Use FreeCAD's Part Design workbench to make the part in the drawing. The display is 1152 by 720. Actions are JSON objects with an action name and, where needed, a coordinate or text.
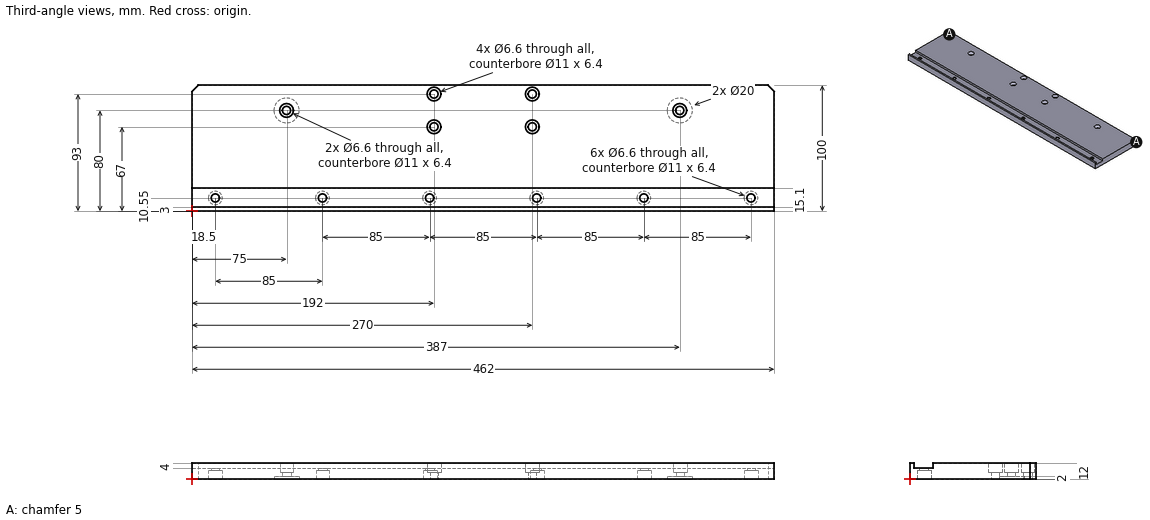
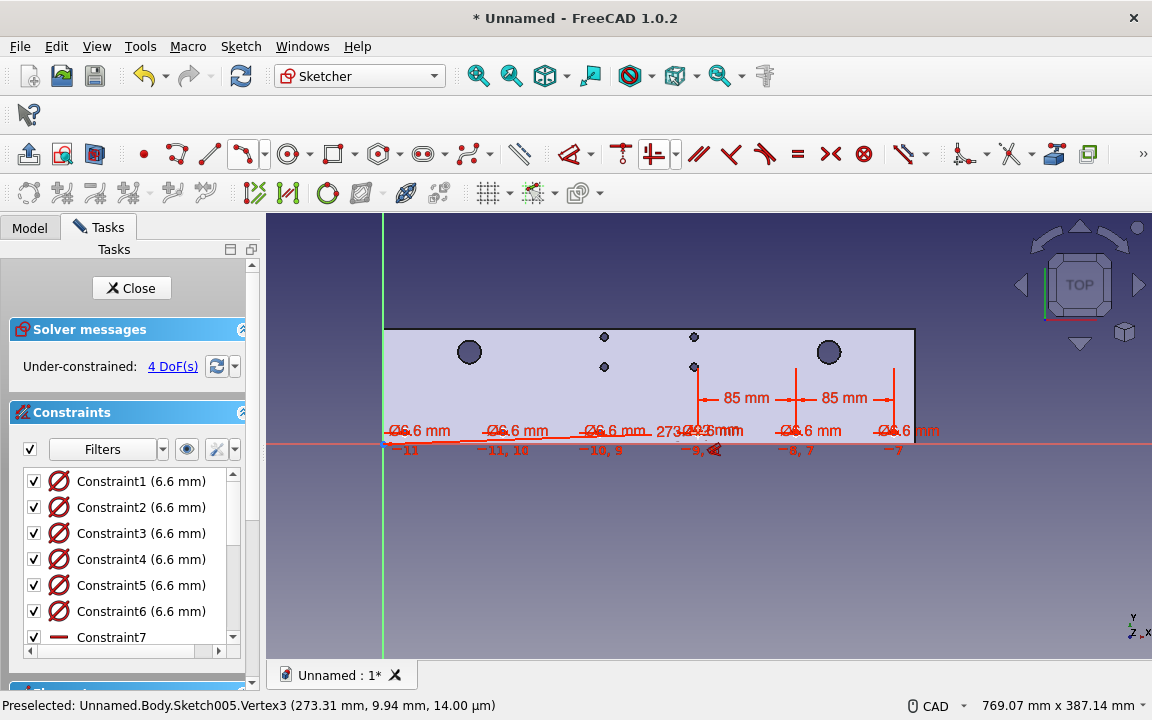
{"action": "left_click", "coordinate": [600, 433]}
{"action": "left_click", "coordinate": [649, 399]}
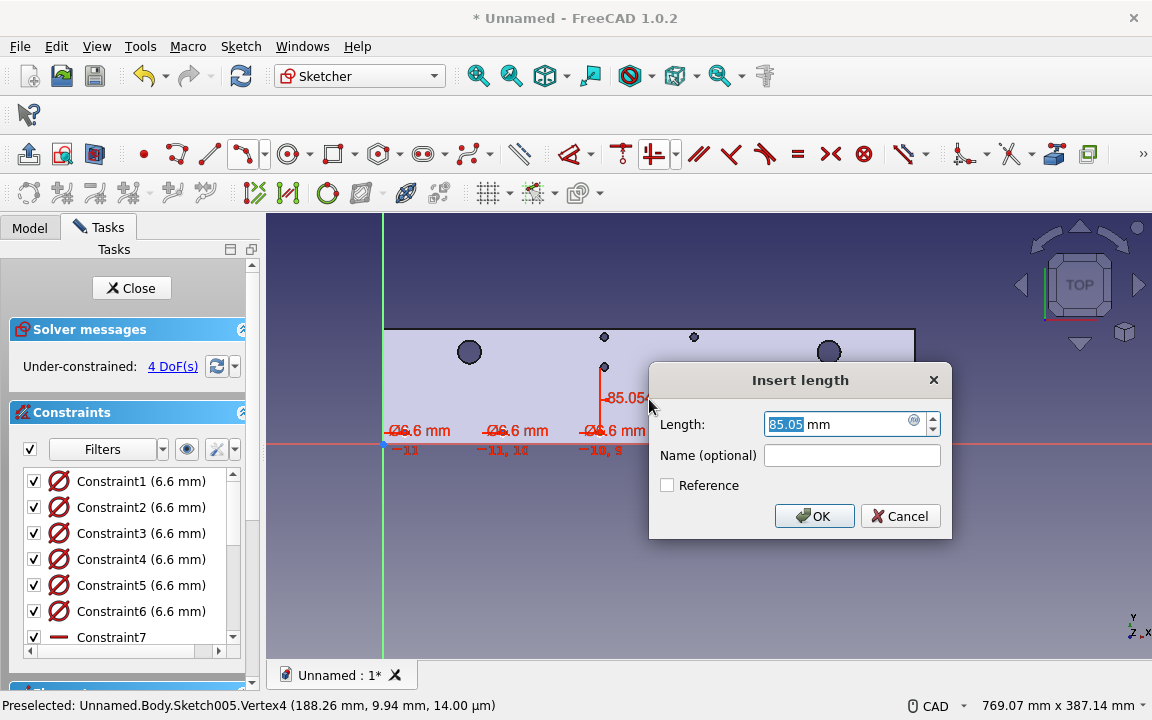
{"action": "type", "text": "85"}
{"action": "key", "text": "Return"}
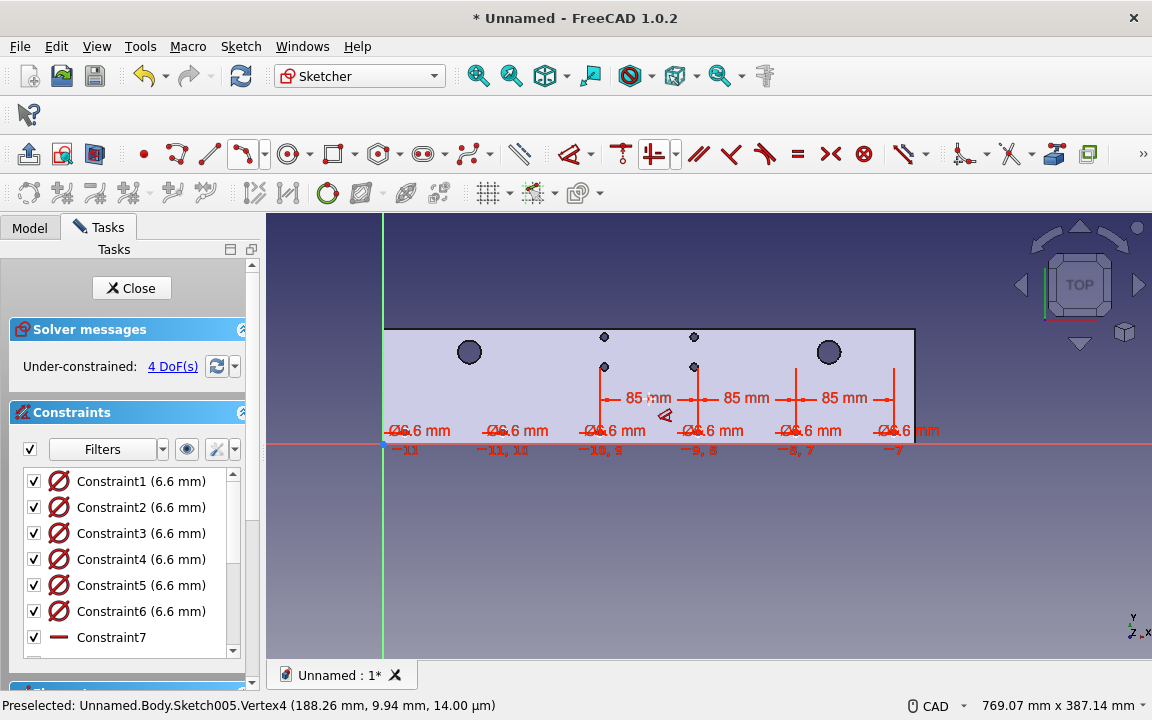
{"action": "left_click", "coordinate": [600, 433]}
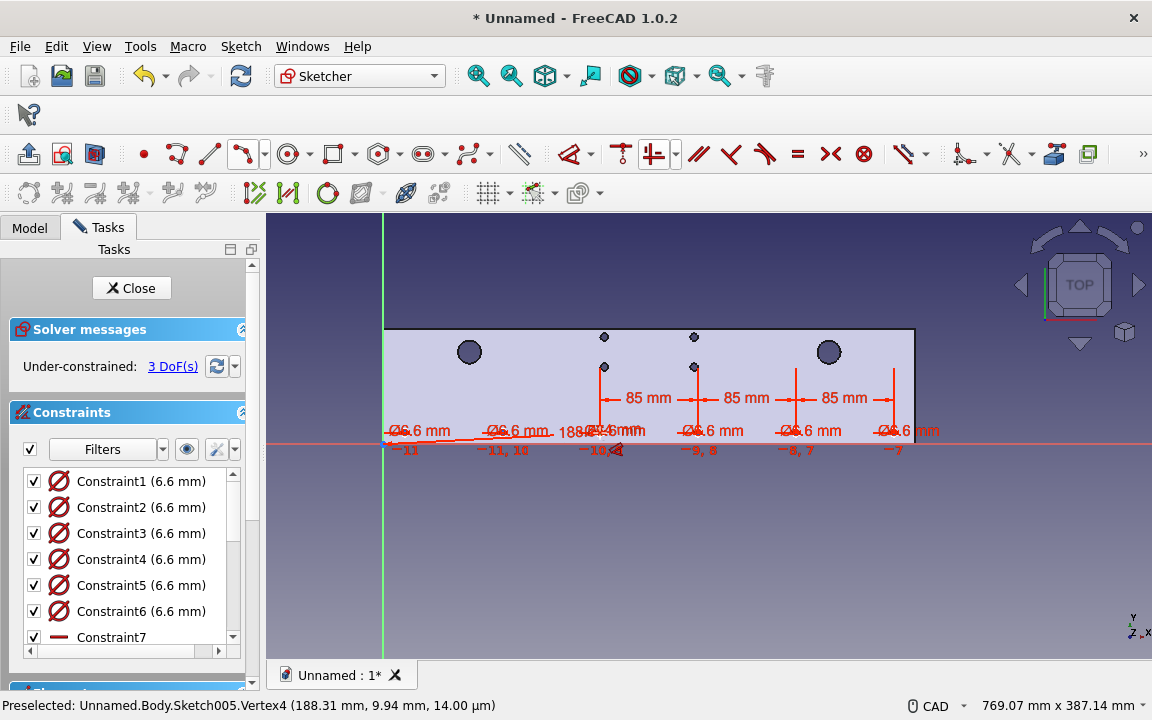
{"action": "left_click", "coordinate": [503, 433]}
{"action": "left_click", "coordinate": [551, 399]}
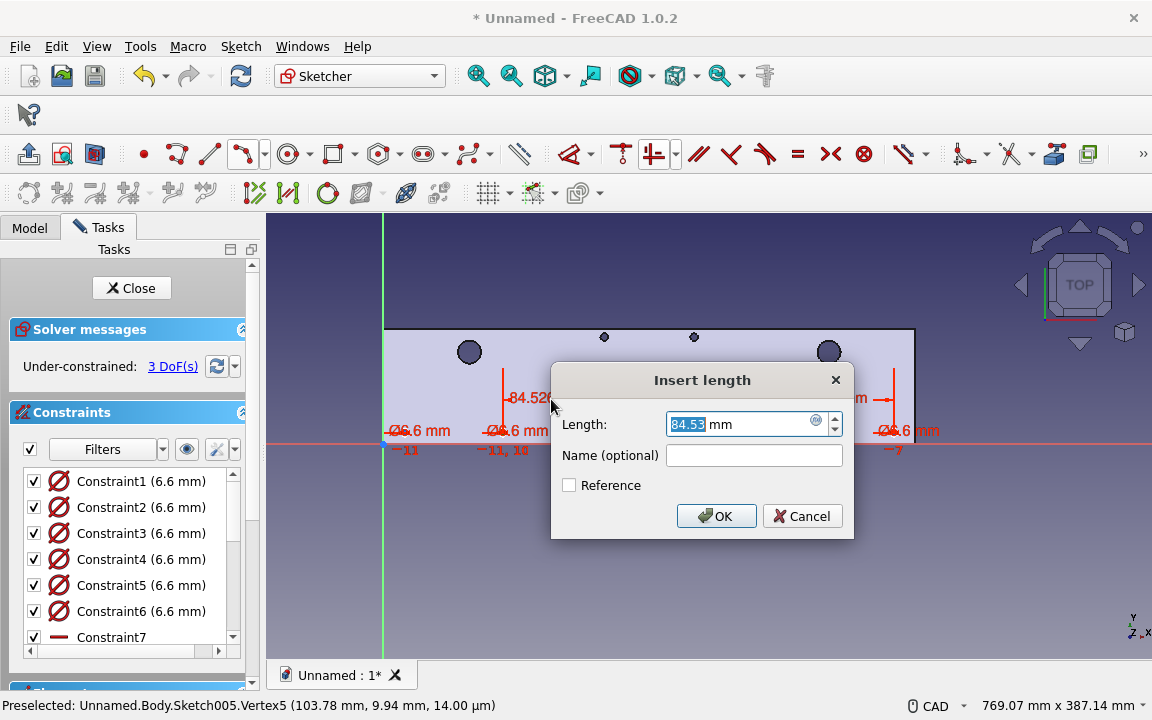
{"action": "type", "text": "85"}
{"action": "key", "text": "Return"}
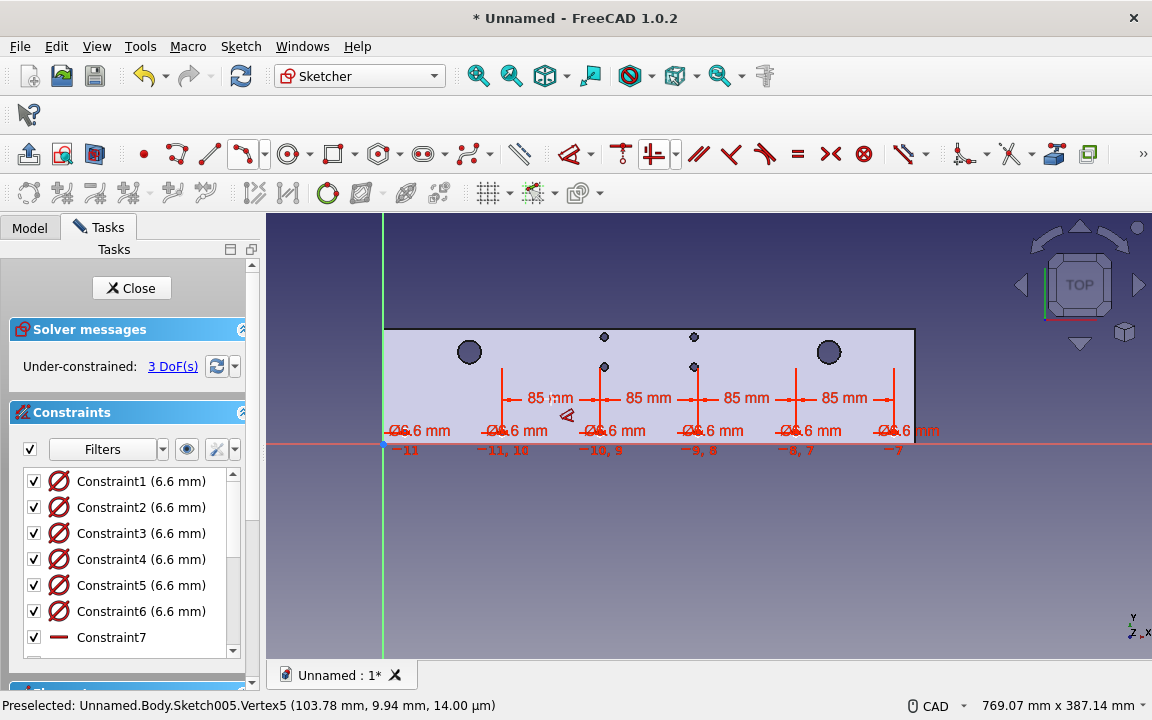
{"action": "left_click", "coordinate": [502, 433]}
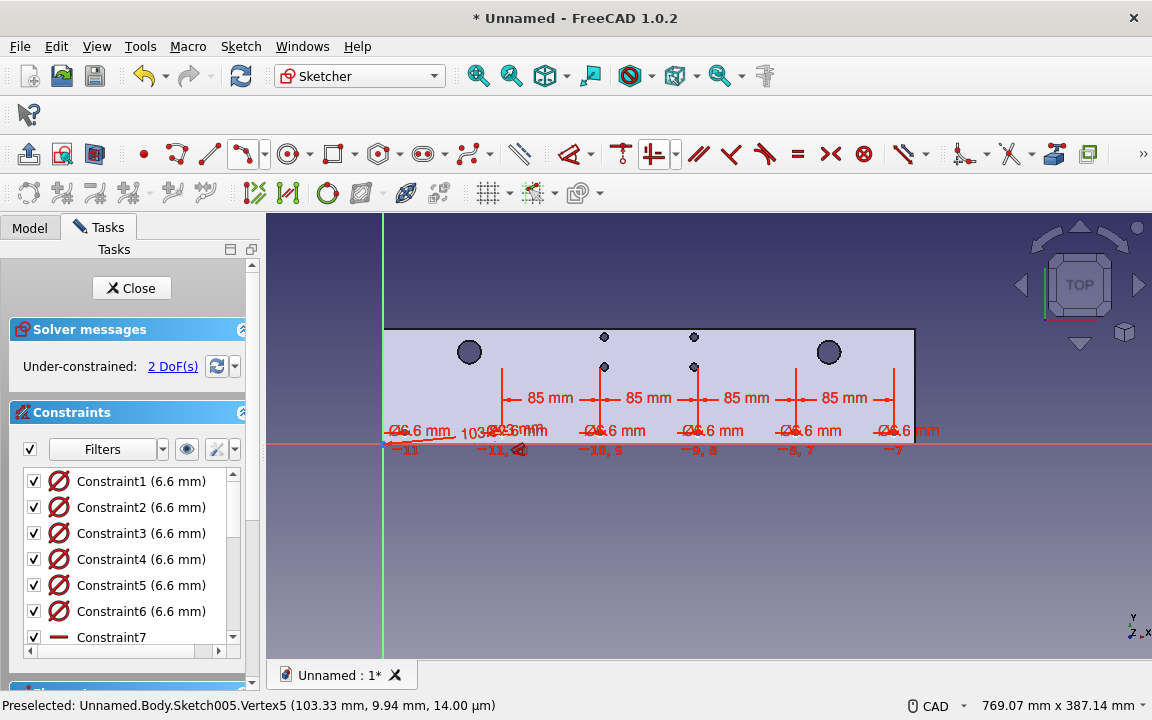
{"action": "left_click", "coordinate": [405, 433]}
{"action": "left_click", "coordinate": [453, 399]}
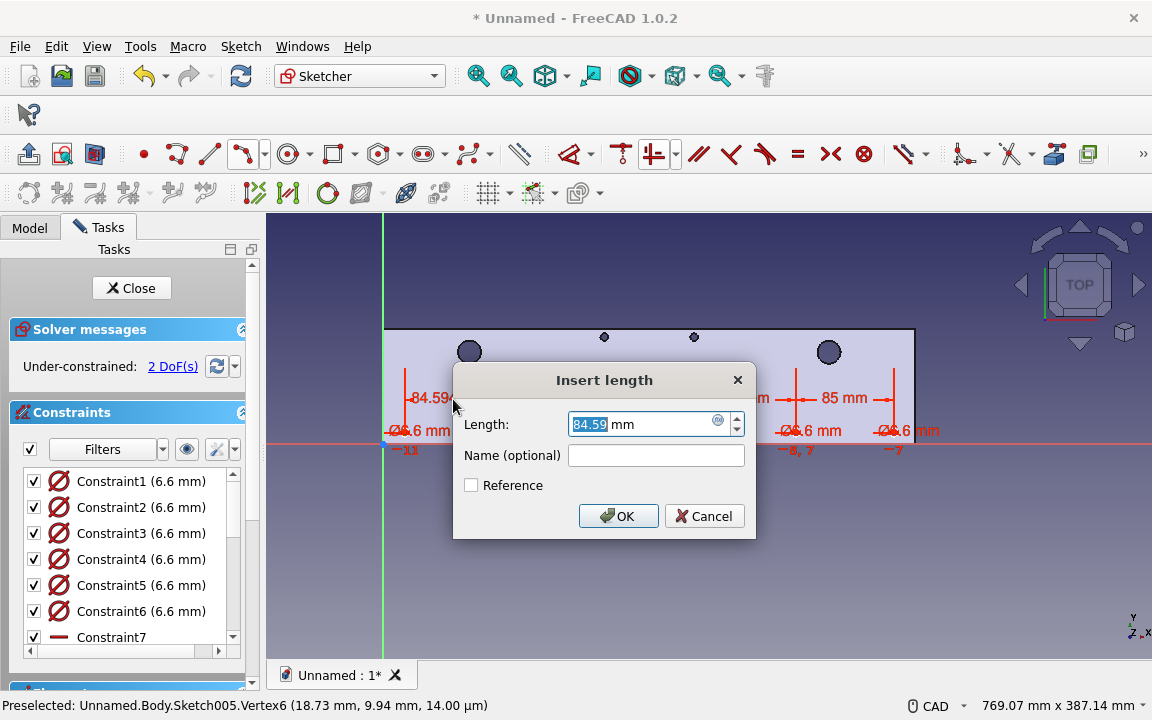
{"action": "type", "text": "85"}
{"action": "key", "text": "Return"}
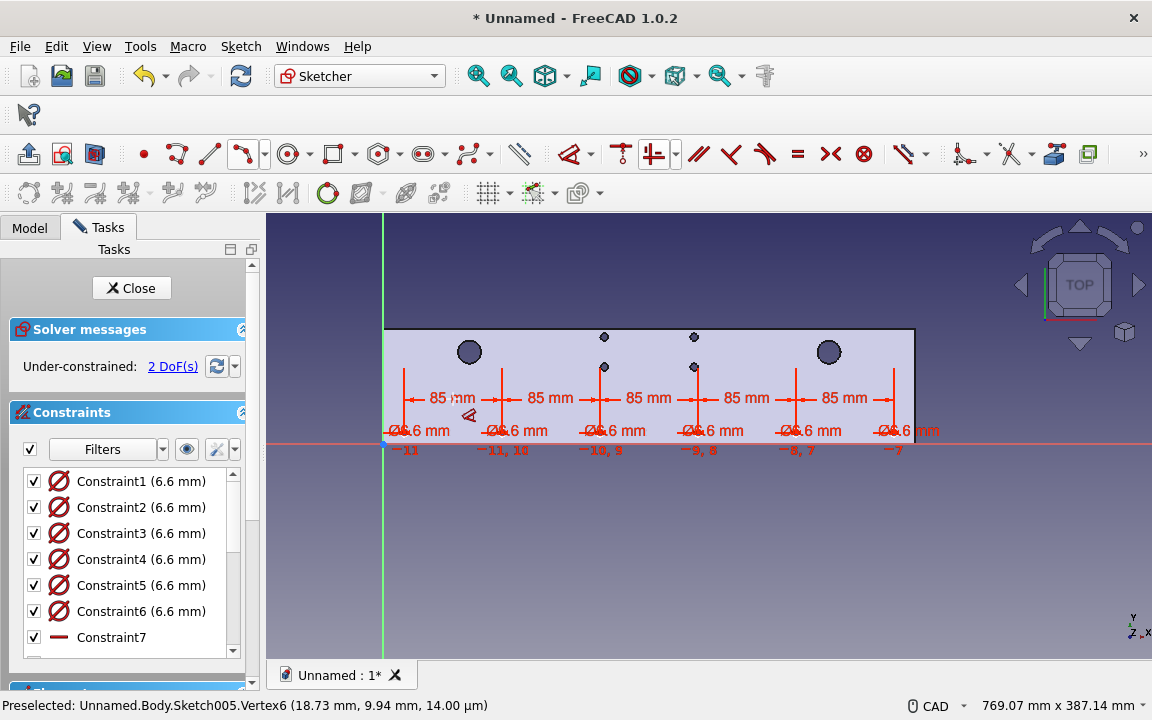
{"action": "scroll", "coordinate": [404, 433], "scroll_direction": "up", "scroll_amount": 4}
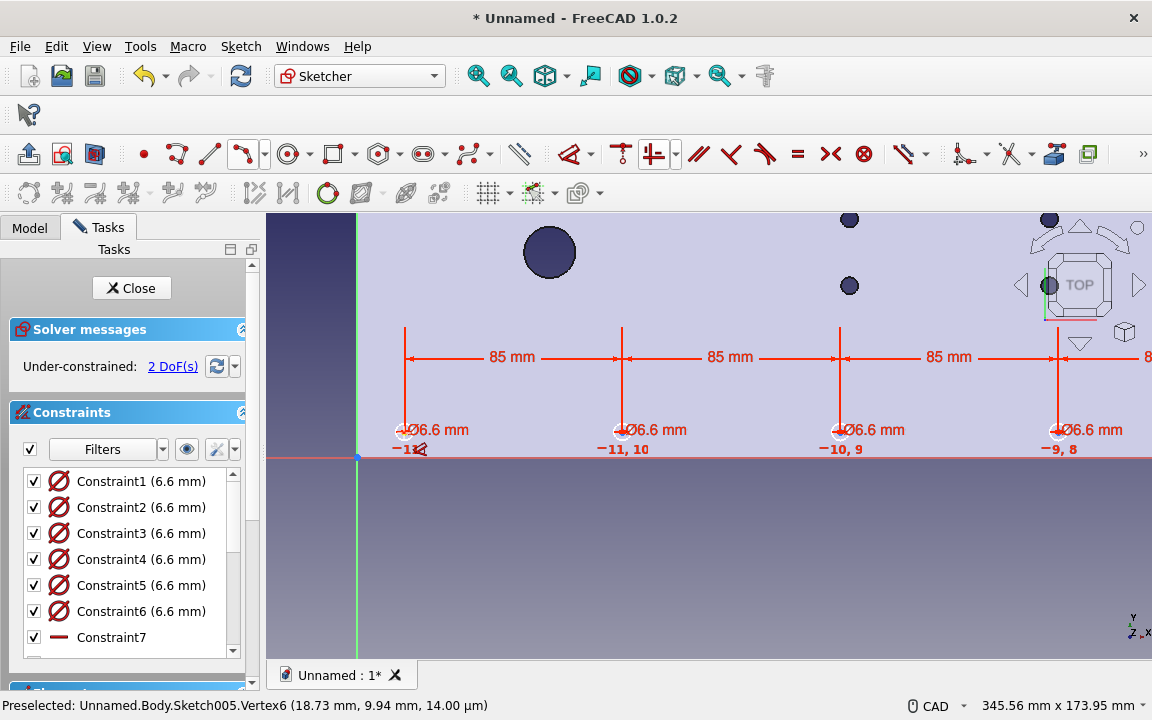
{"action": "left_click", "coordinate": [405, 432]}
{"action": "left_click", "coordinate": [381, 492]}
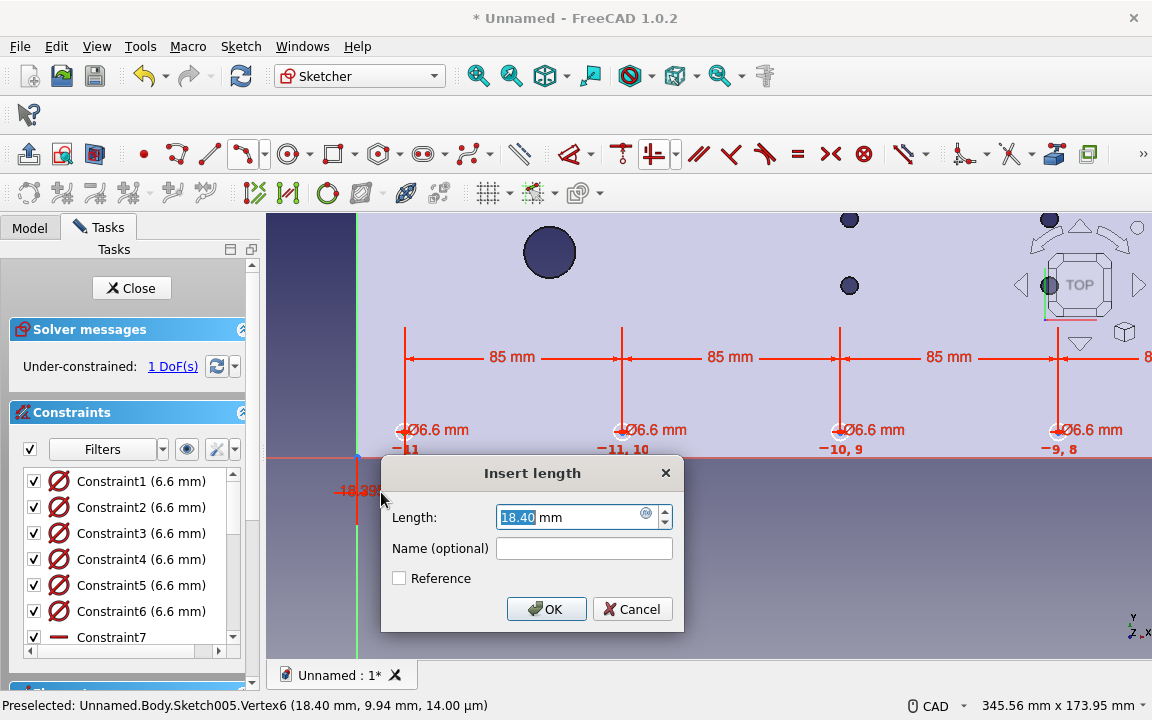
{"action": "type", "text": "18.5"}
{"action": "key", "text": "Return"}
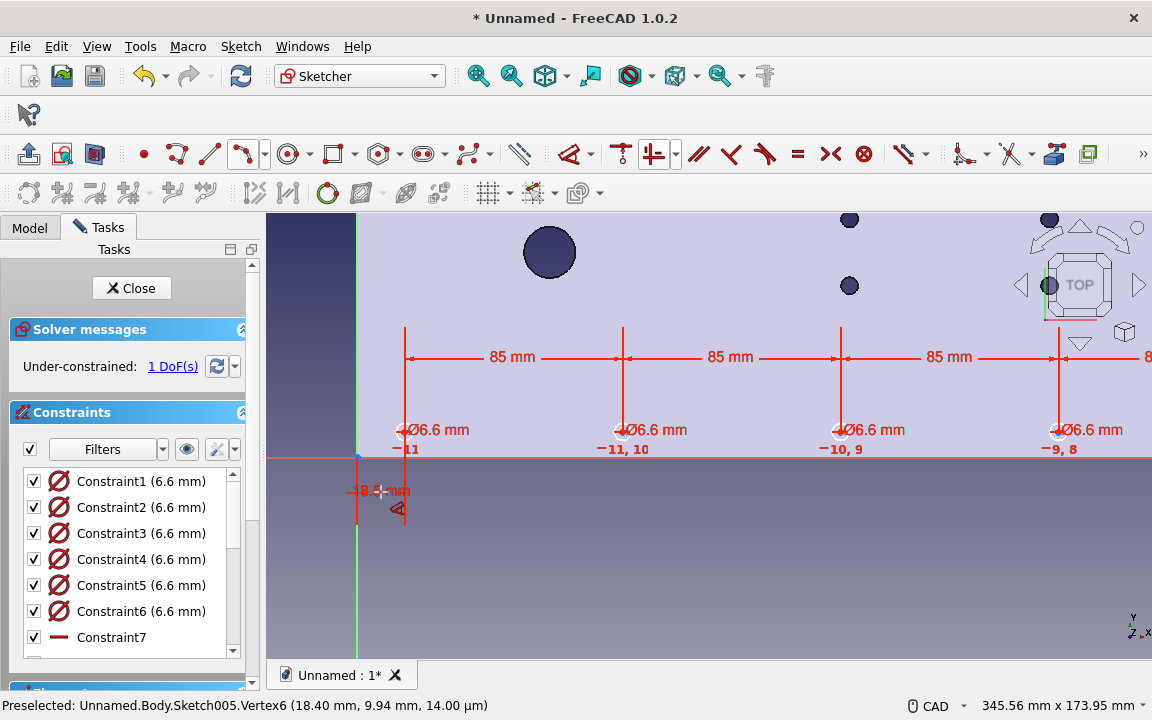
{"action": "scroll", "coordinate": [404, 433], "scroll_direction": "down", "scroll_amount": 4}